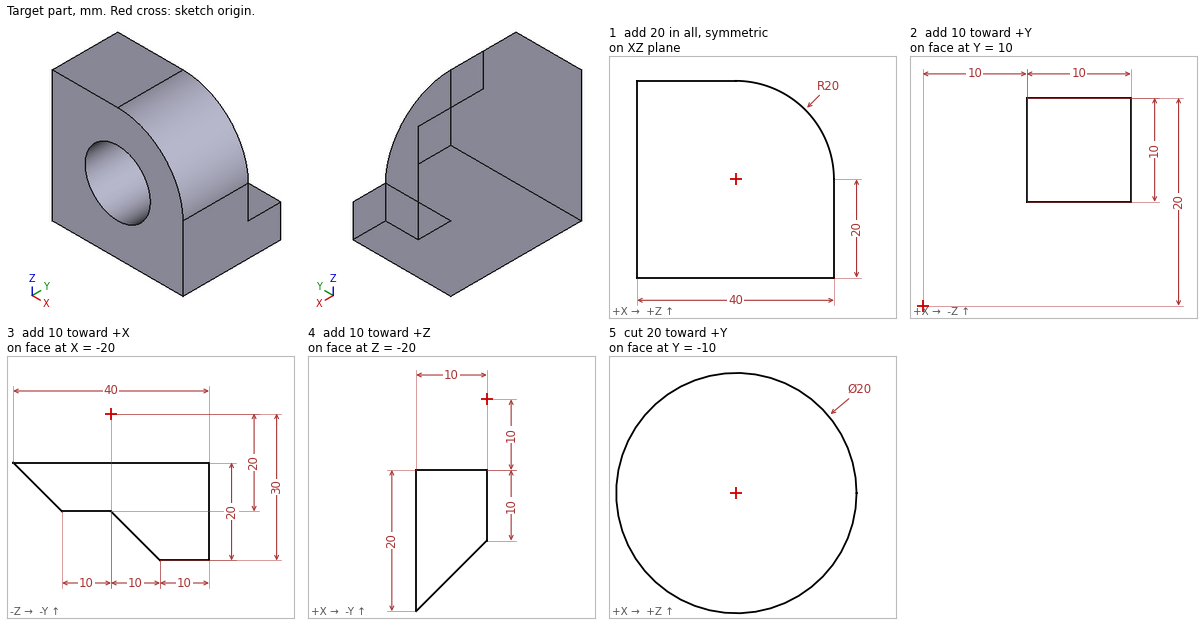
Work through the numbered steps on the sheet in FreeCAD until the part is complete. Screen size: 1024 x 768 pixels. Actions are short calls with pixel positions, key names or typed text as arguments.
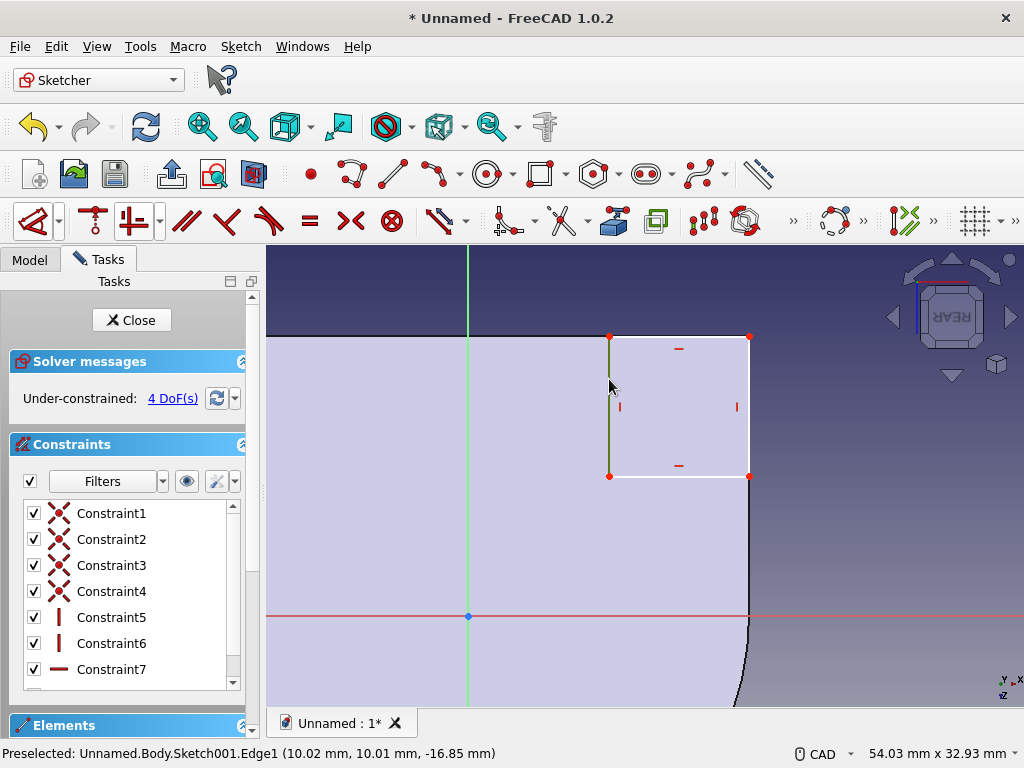
click(58, 222)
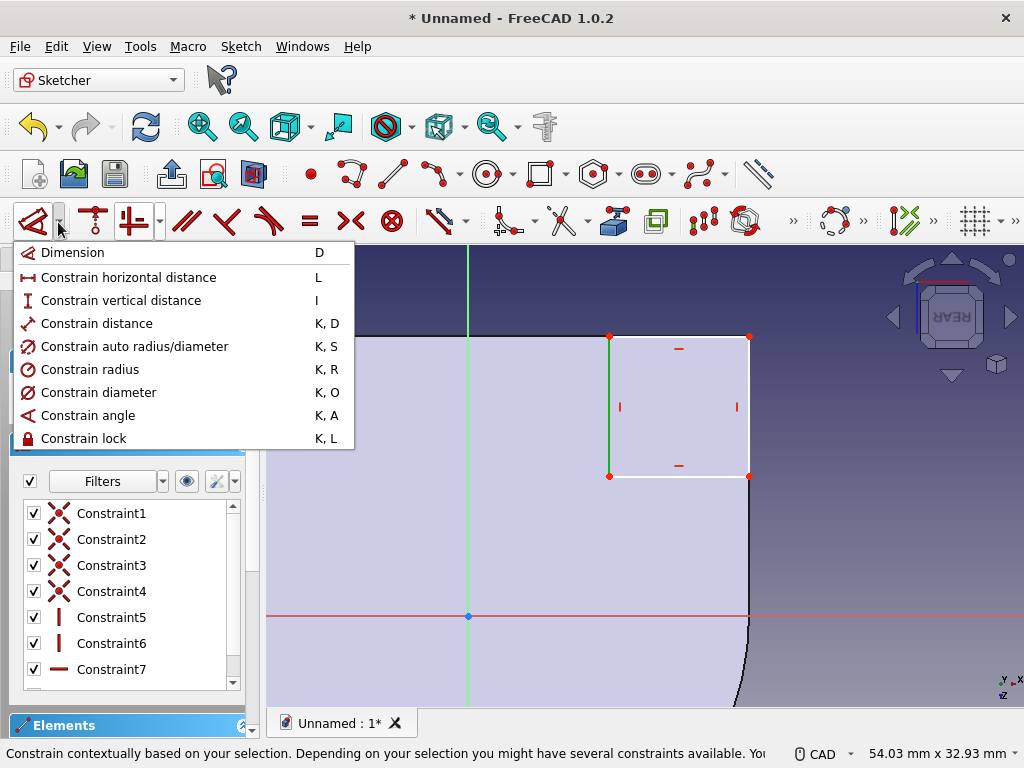
click(184, 300)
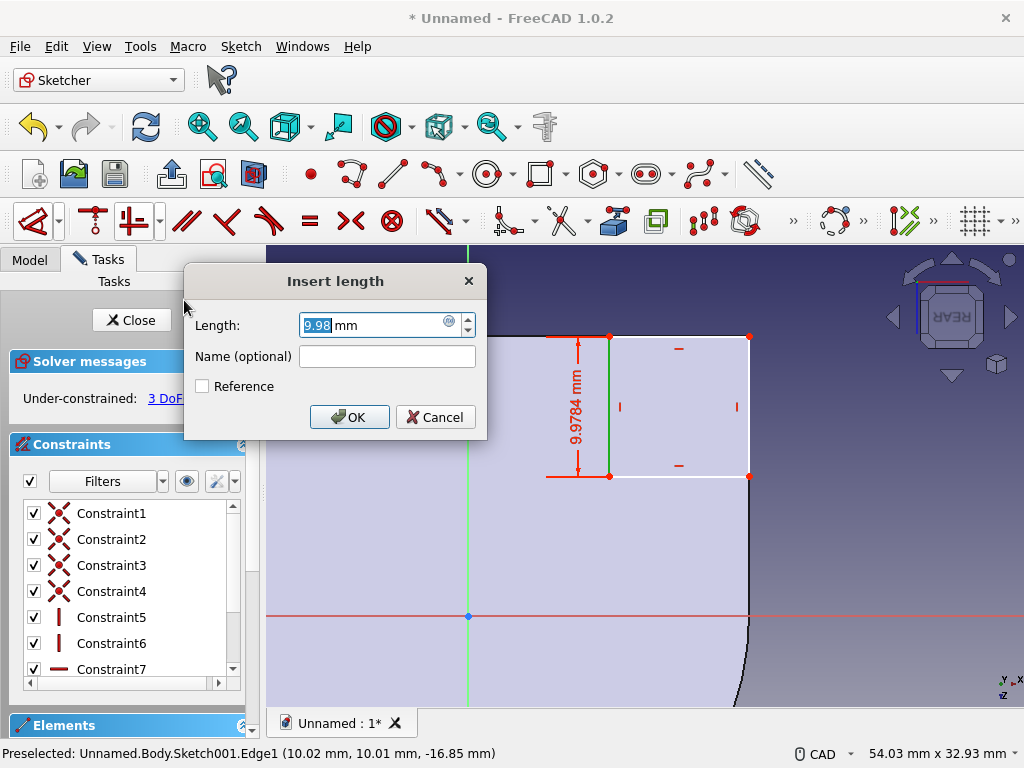
text(10)
key(Return)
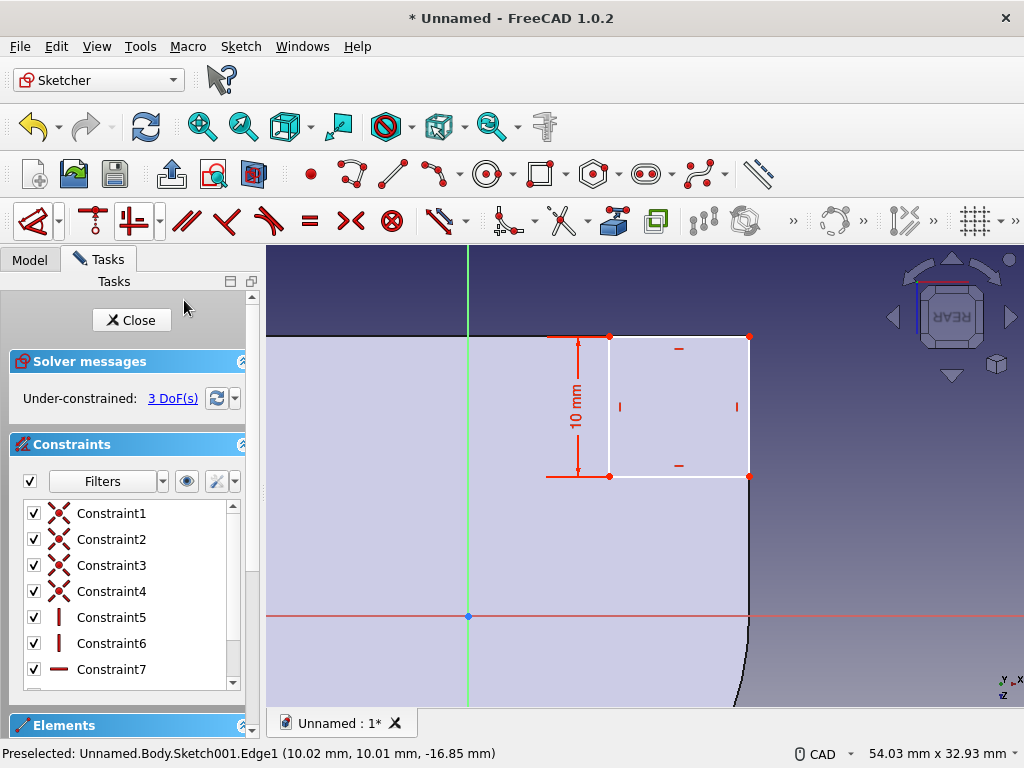
click(651, 477)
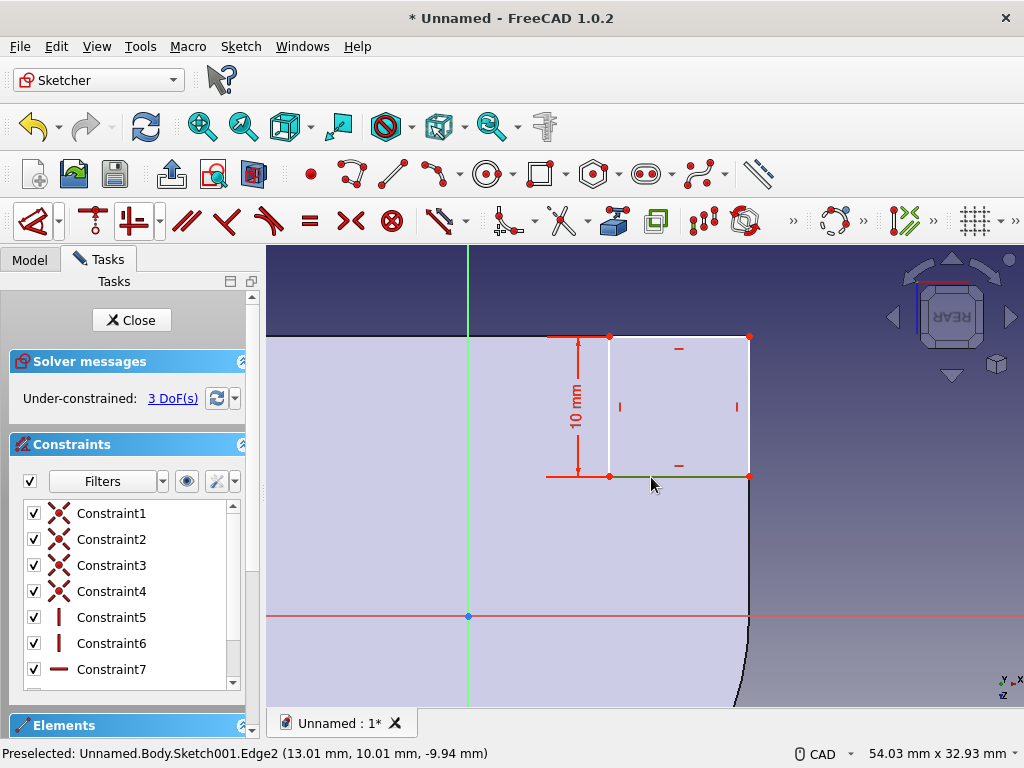
click(58, 222)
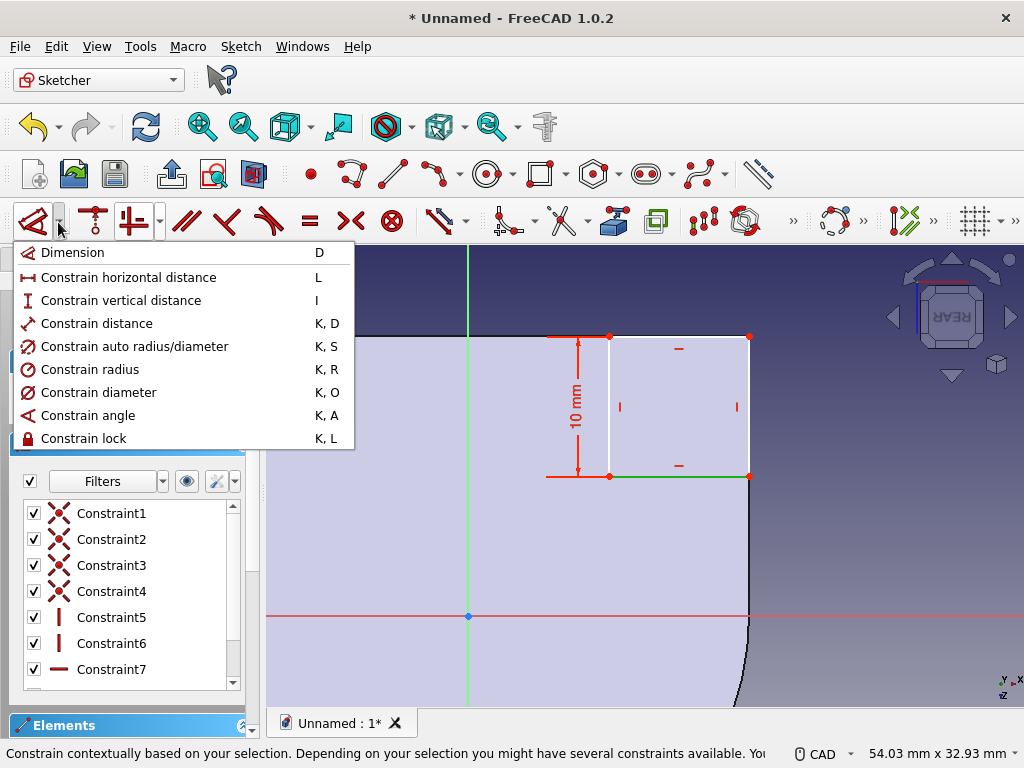
click(184, 278)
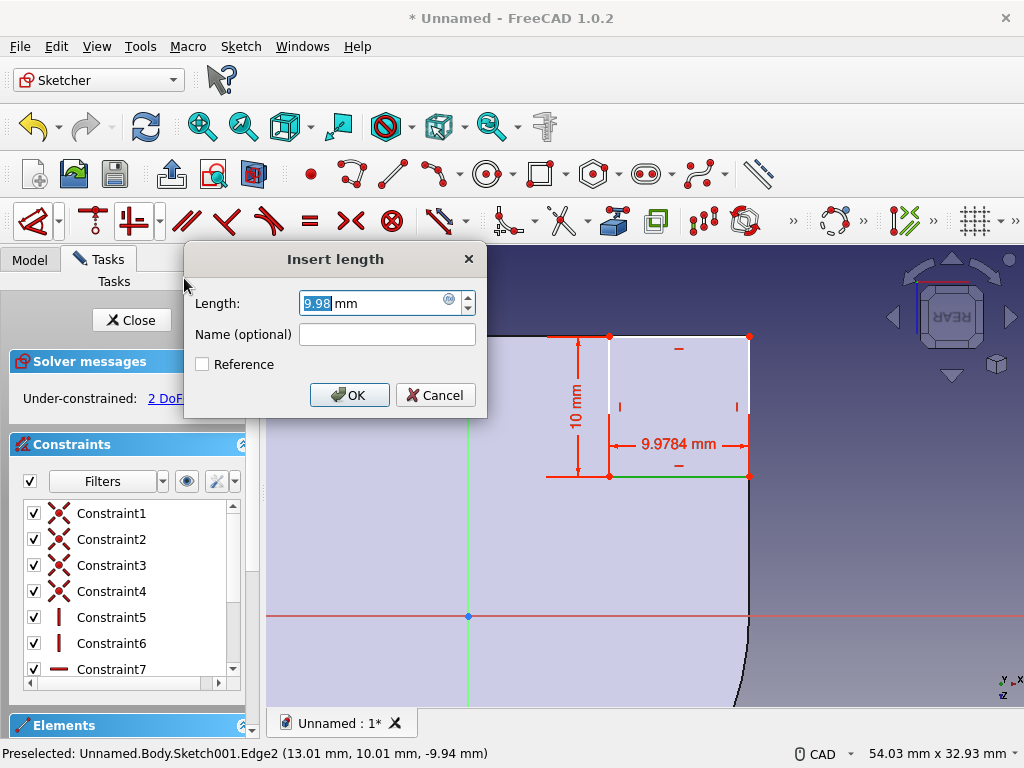
text(10)
key(Return)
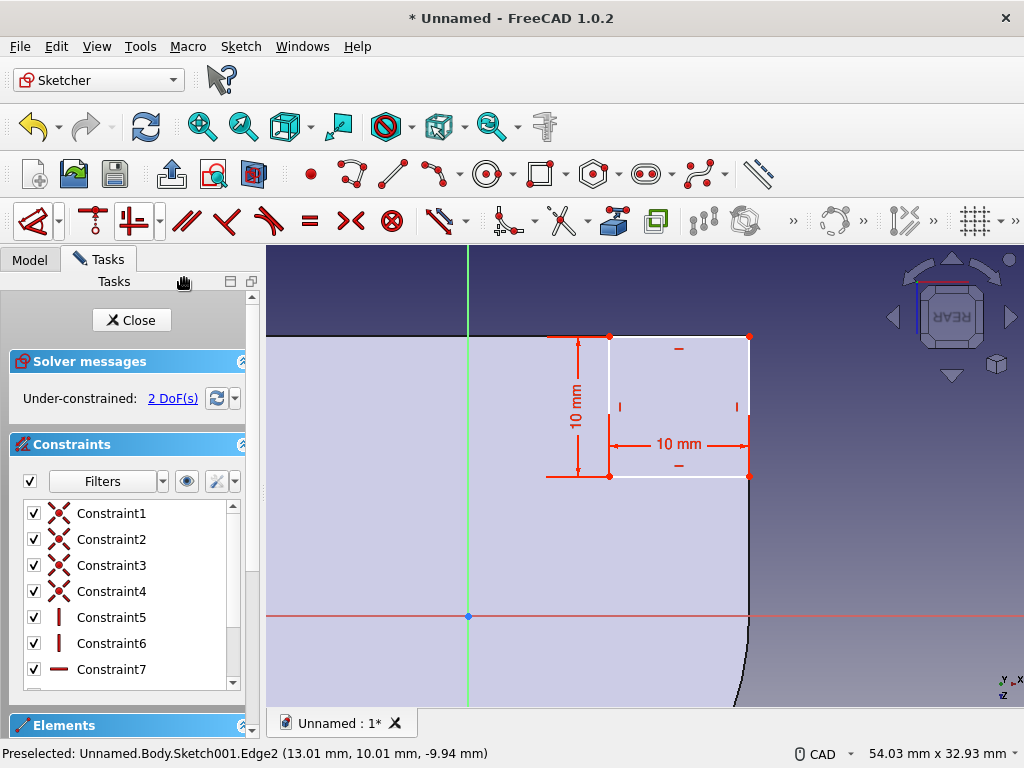
click(609, 337)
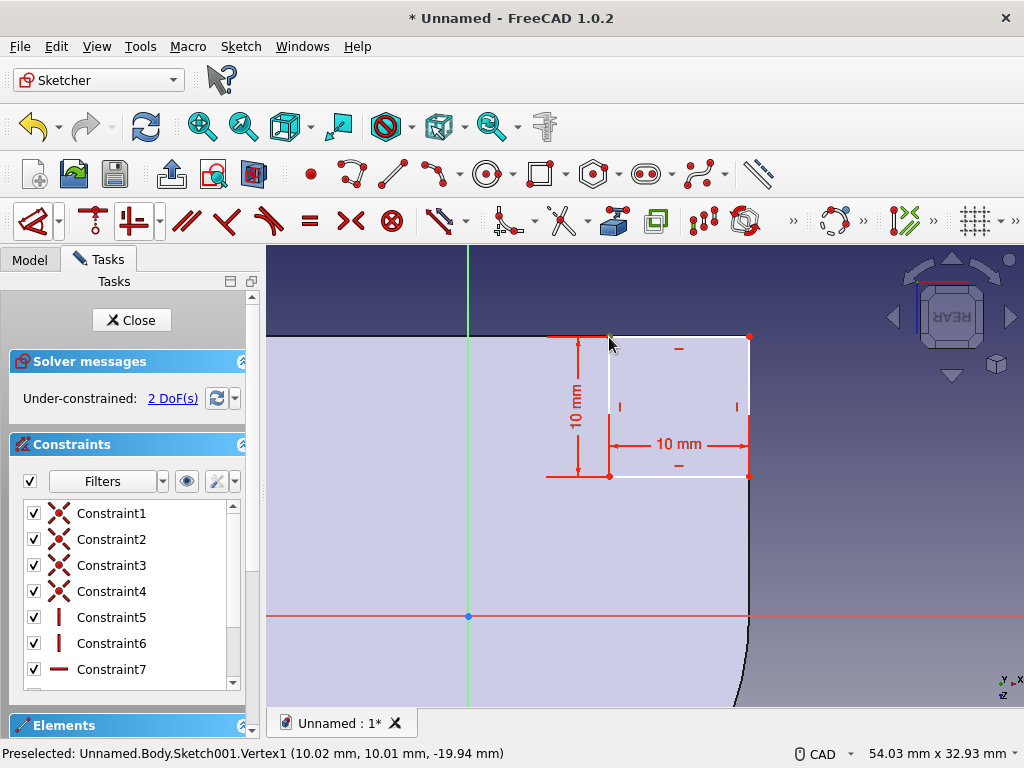
key(l)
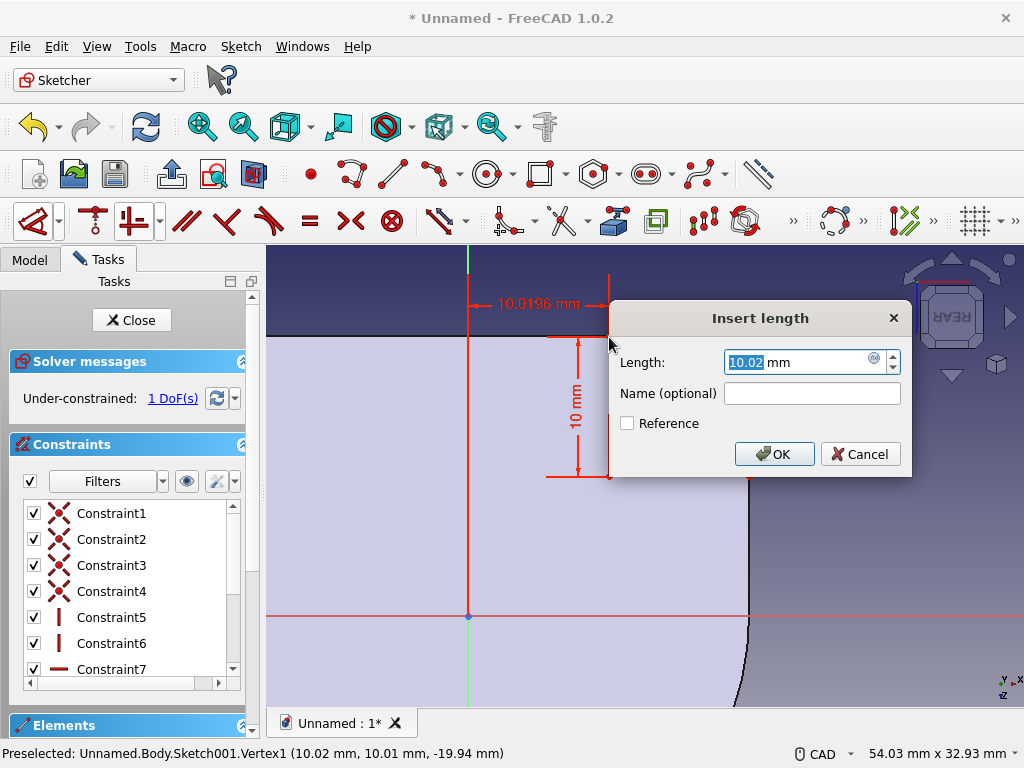
text(10)
key(Return)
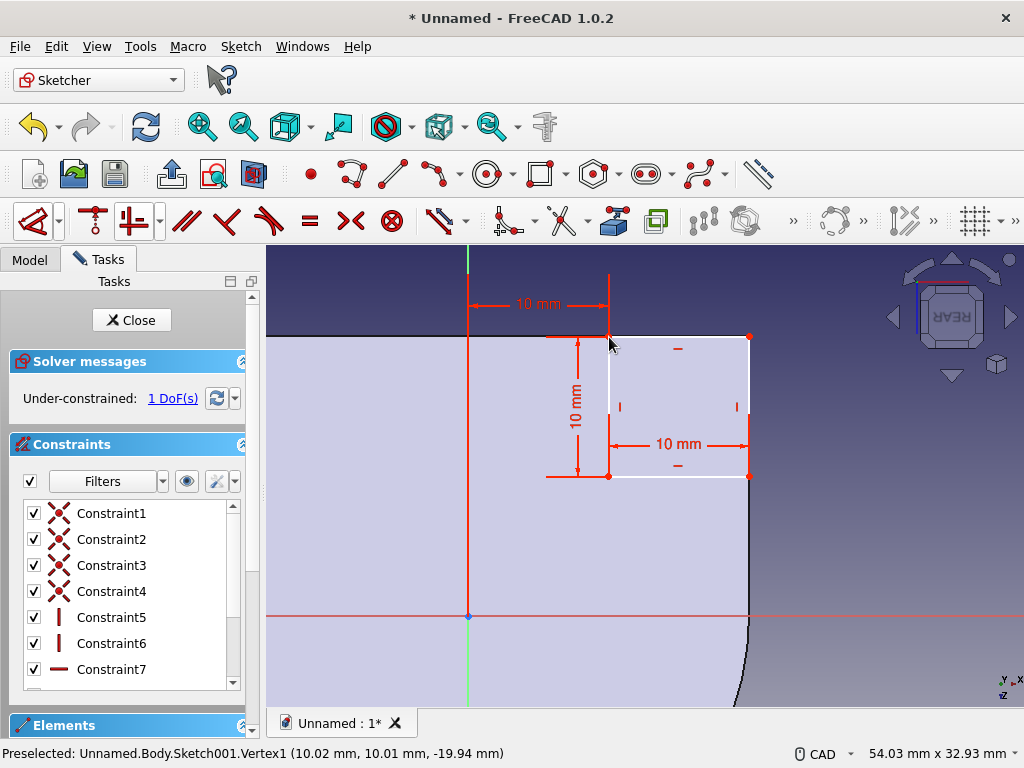
click(609, 337)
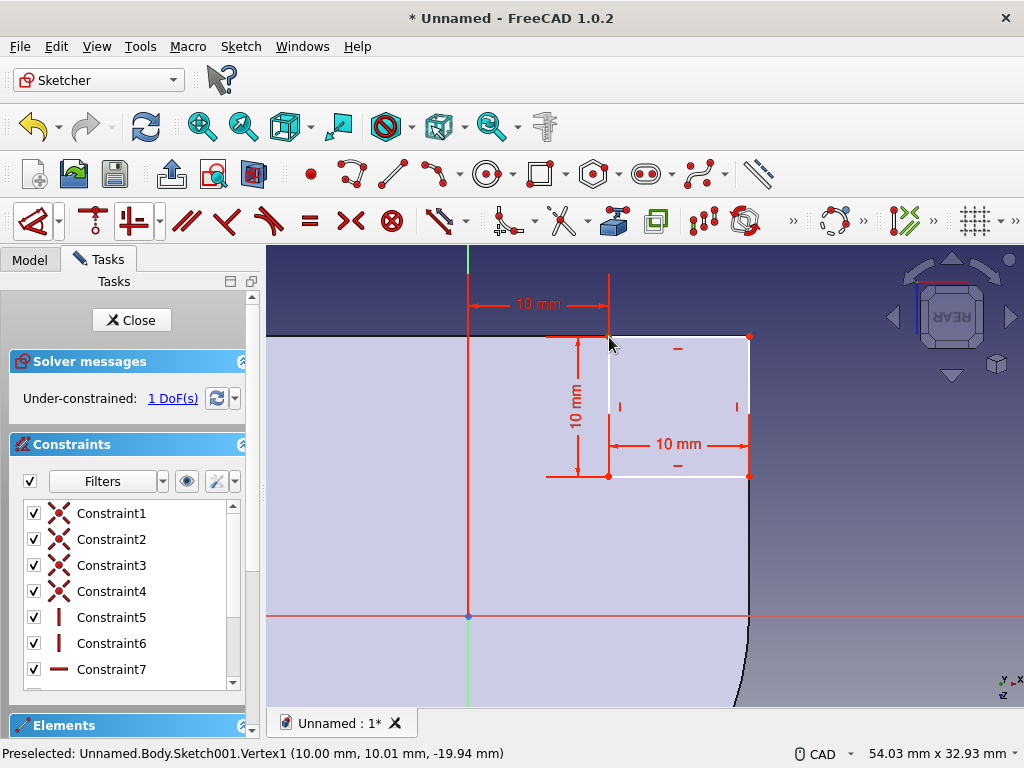
key(i)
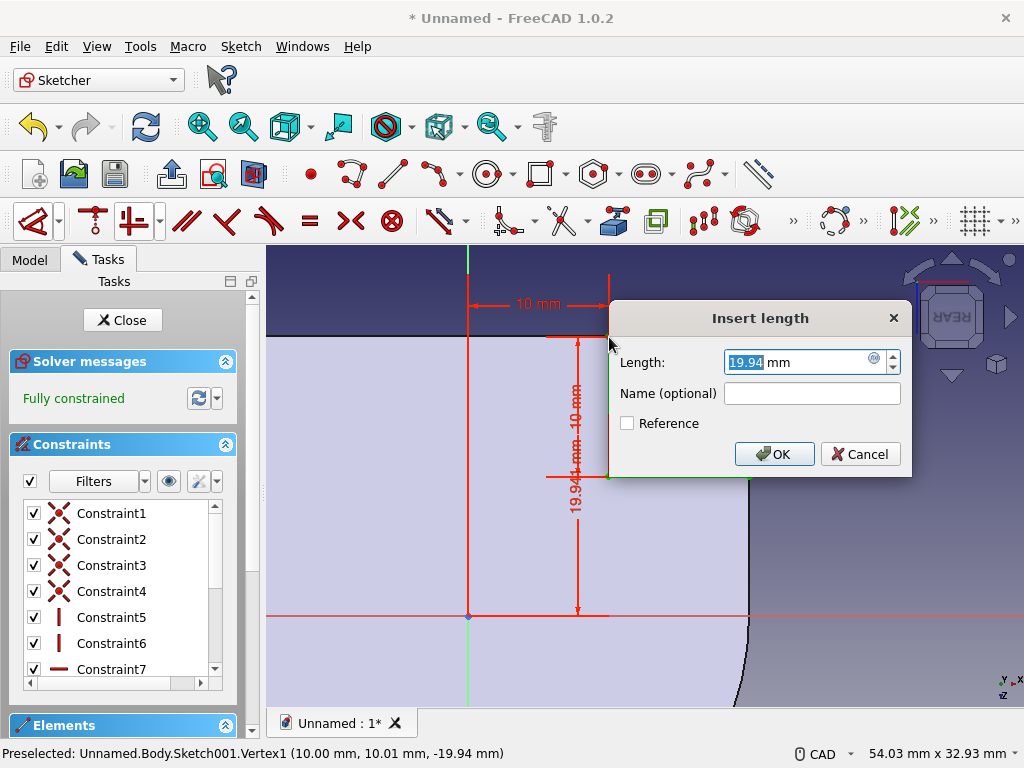
text(20)
key(Return)